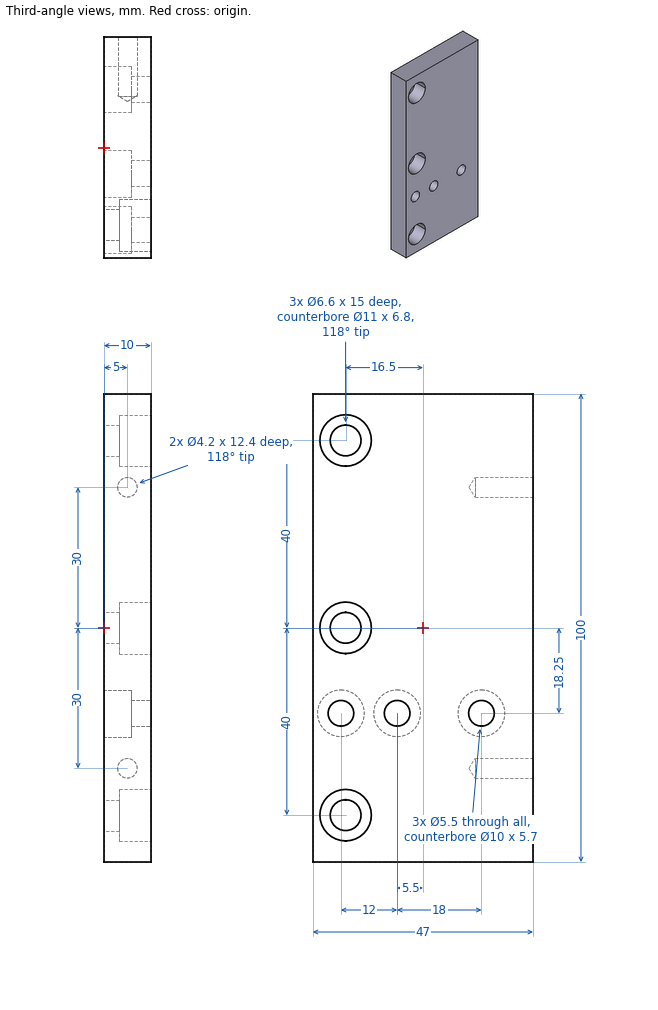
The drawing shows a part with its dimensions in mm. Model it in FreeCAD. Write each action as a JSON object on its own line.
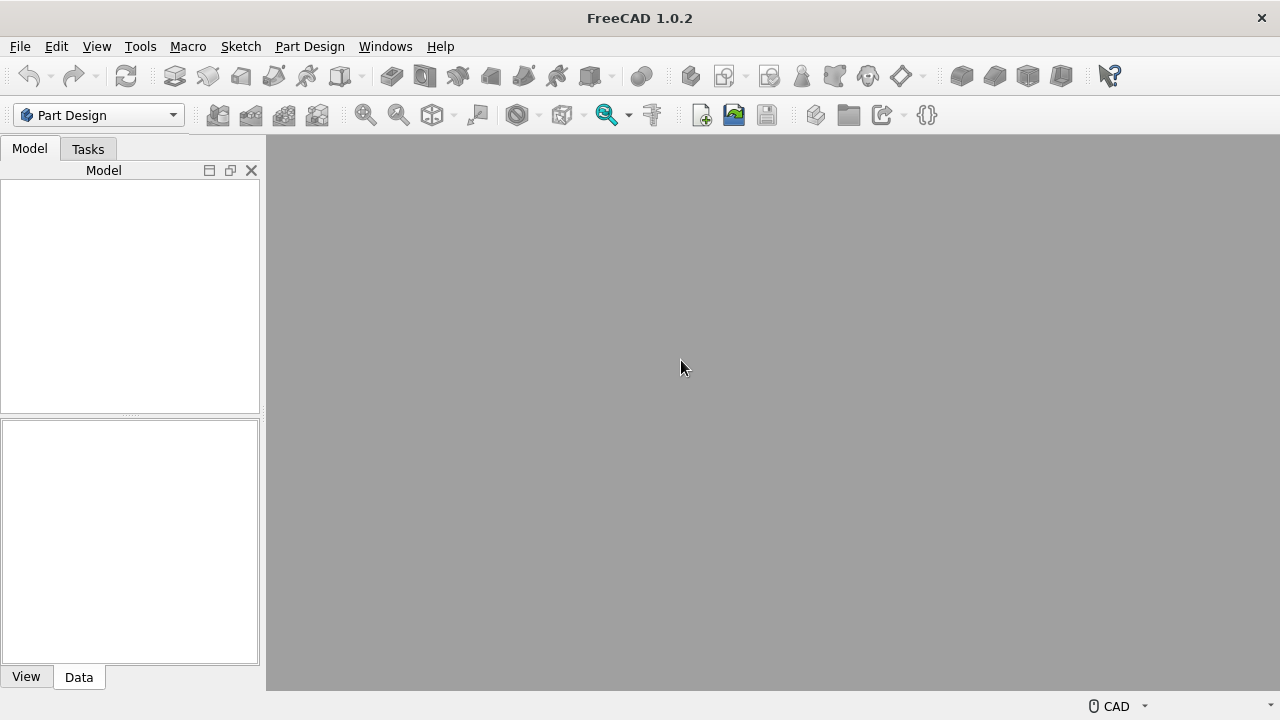
{"action": "left_click", "coordinate": [701, 116]}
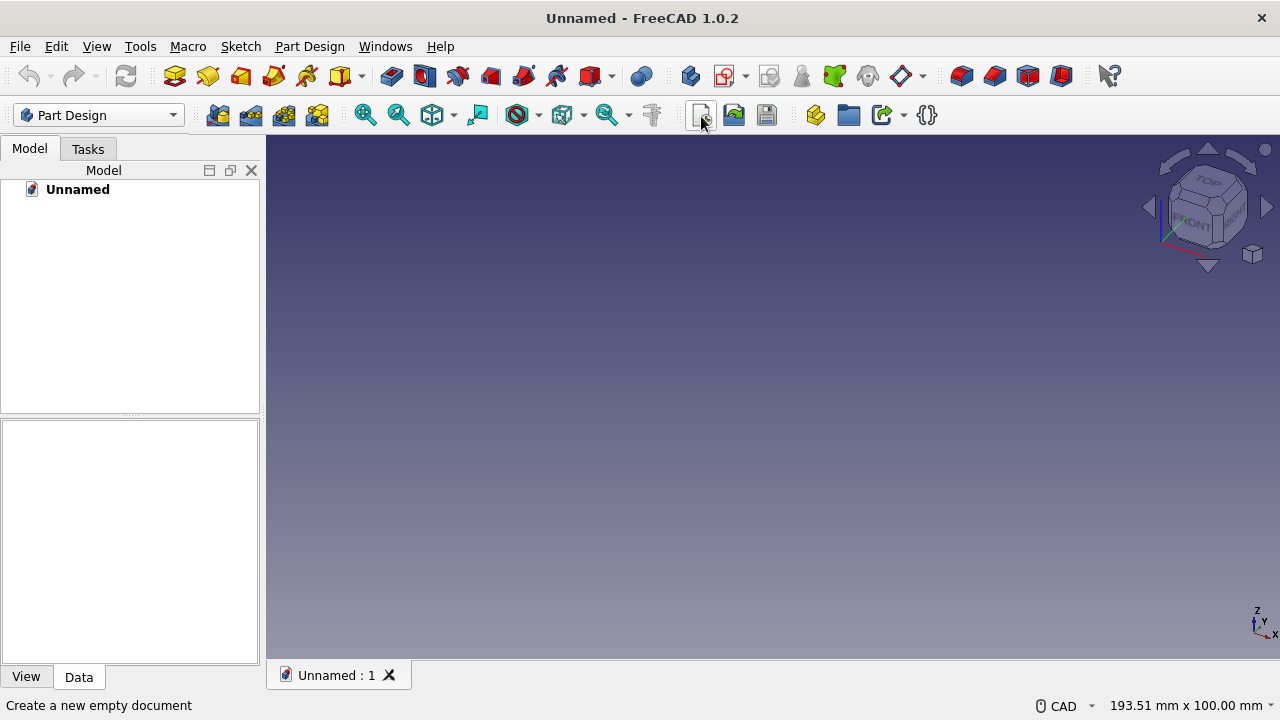
{"action": "left_click", "coordinate": [724, 76]}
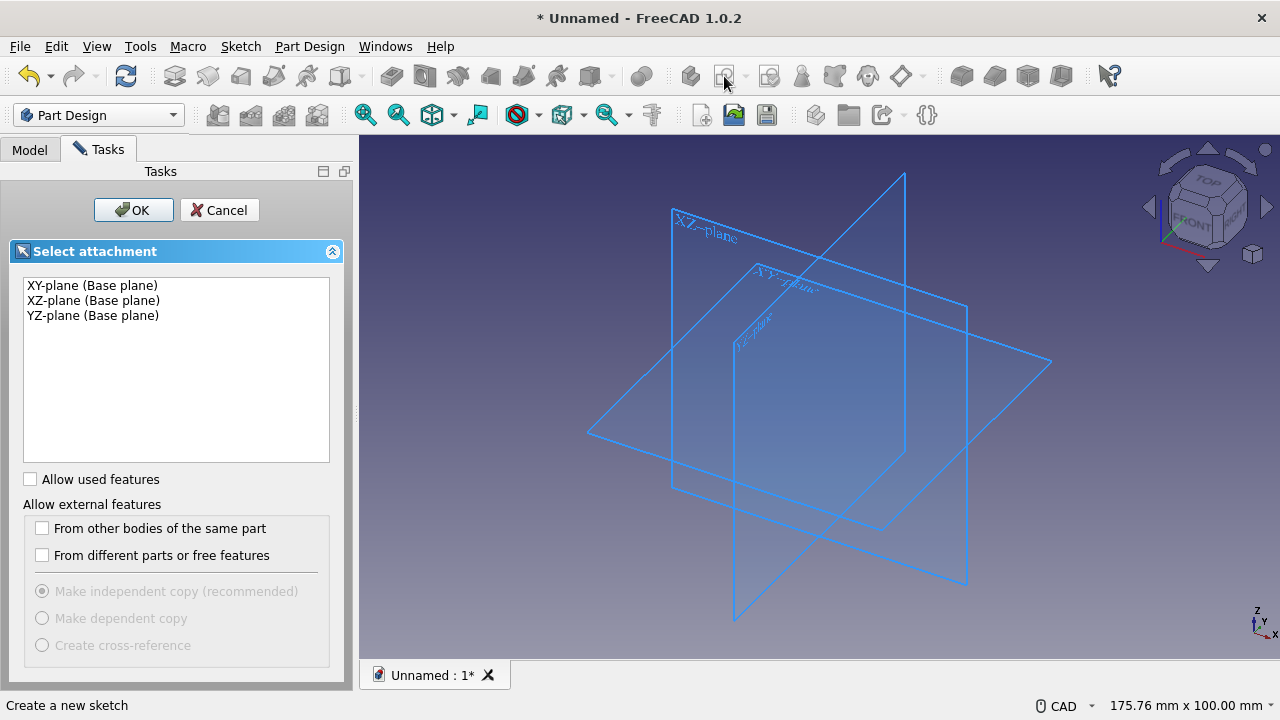
{"action": "left_click", "coordinate": [84, 316]}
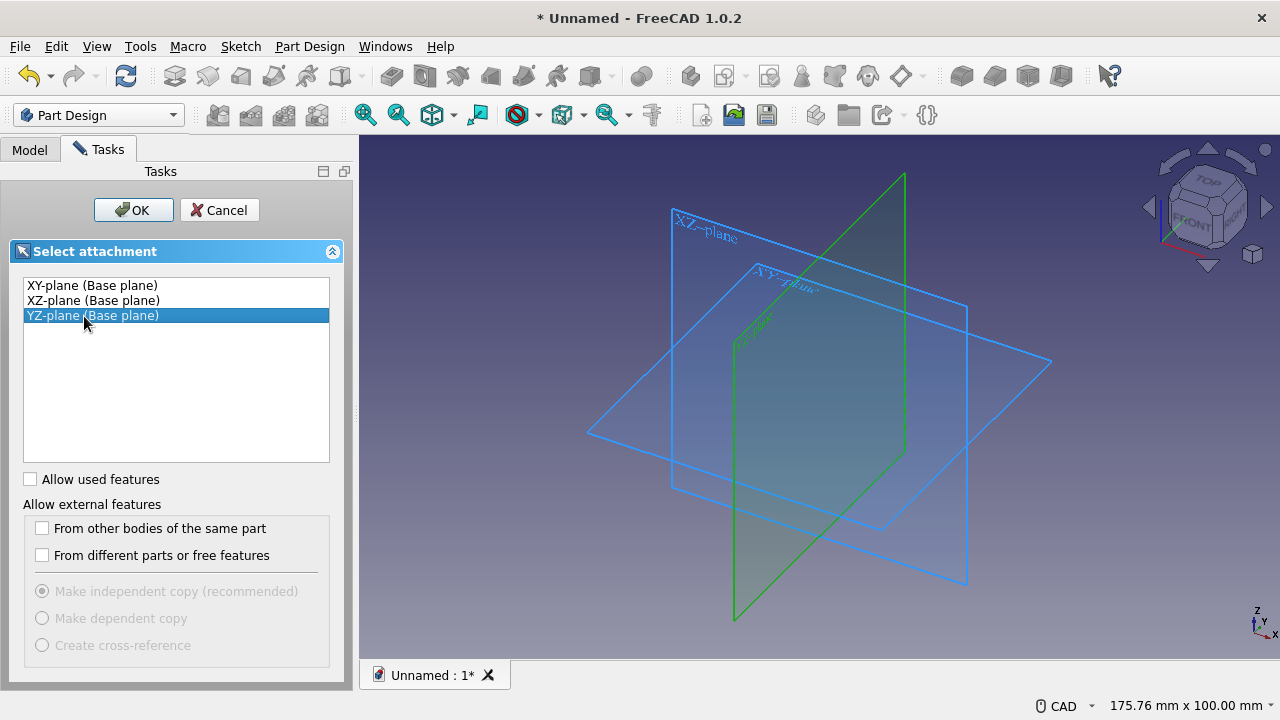
{"action": "left_click", "coordinate": [134, 210]}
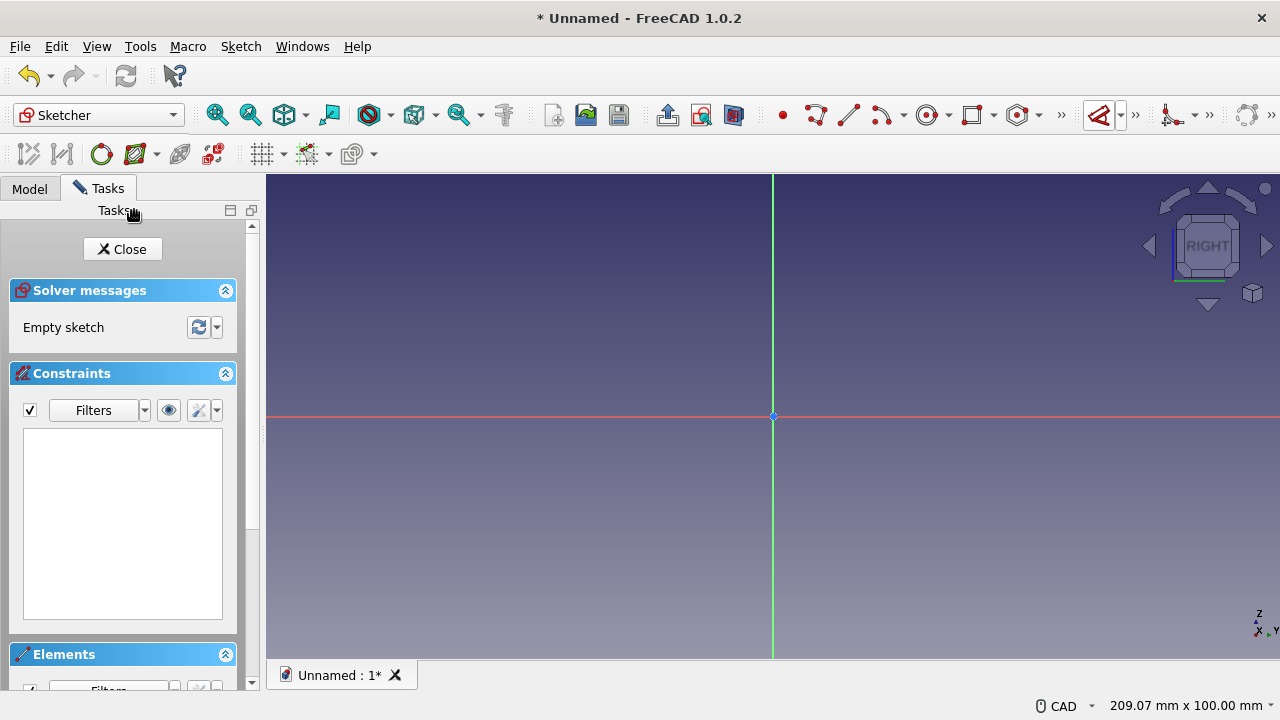
{"action": "scroll", "coordinate": [565, 416], "scroll_direction": "down", "scroll_amount": 2}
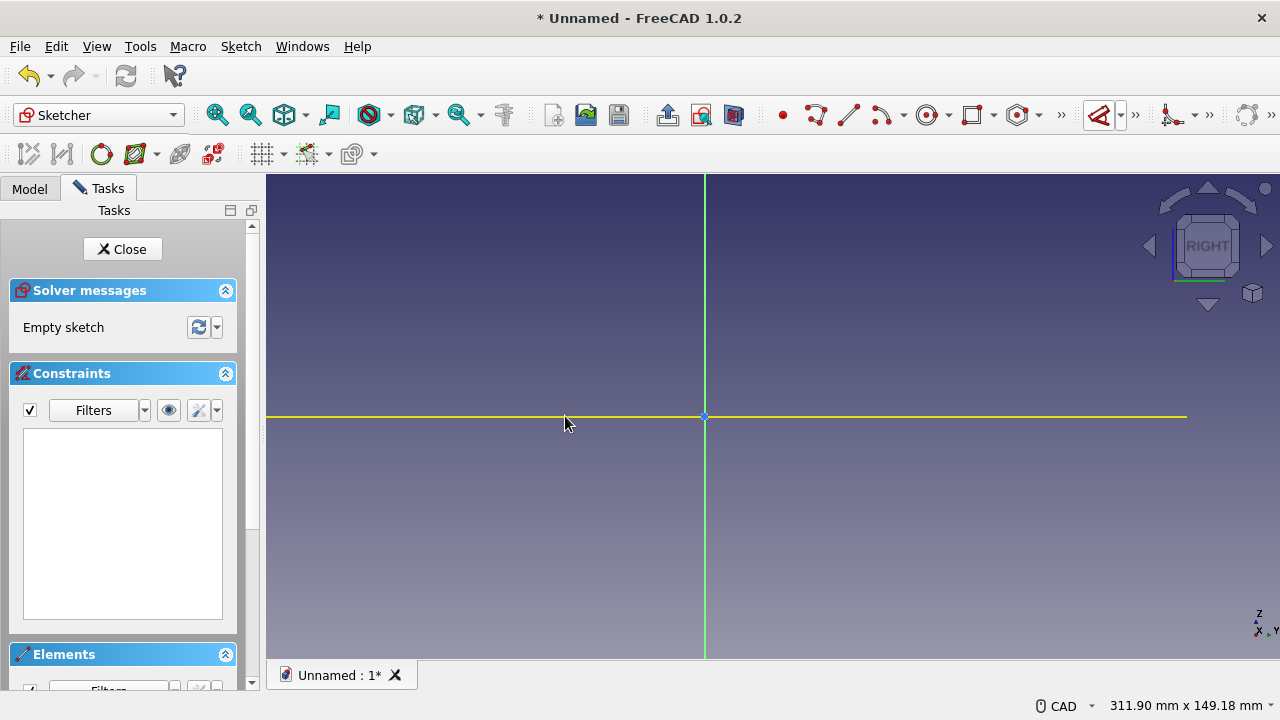
{"action": "key", "text": "g v"}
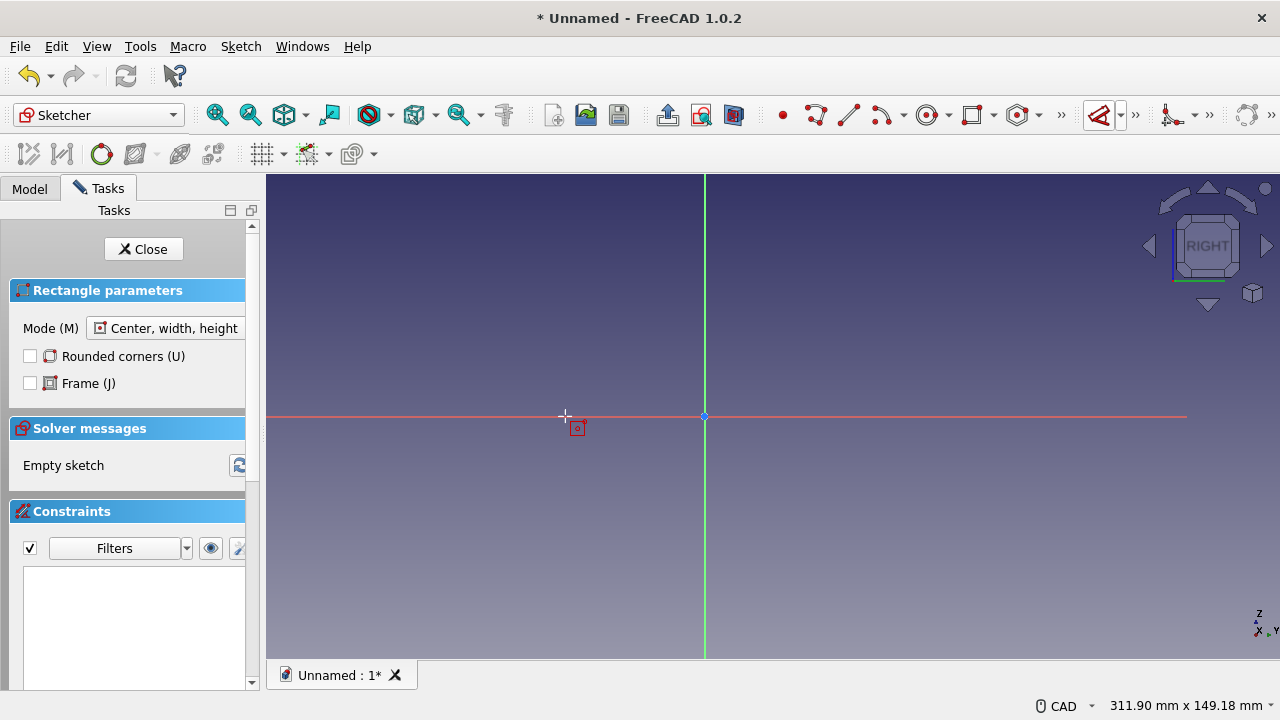
{"action": "left_click", "coordinate": [705, 416]}
{"action": "mouse_move", "coordinate": [781, 254]}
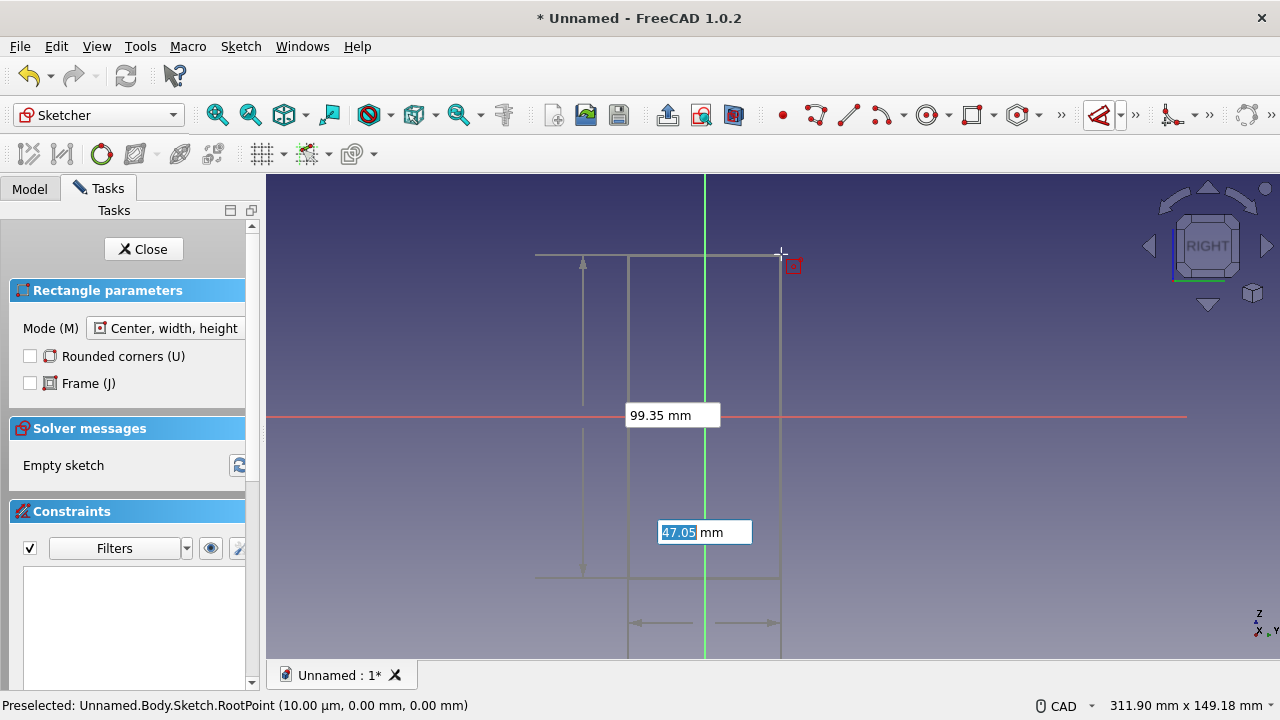
{"action": "type", "text": "47"}
{"action": "key", "text": "Tab"}
{"action": "type", "text": "100"}
{"action": "key", "text": "Return"}
{"action": "key", "text": "Escape"}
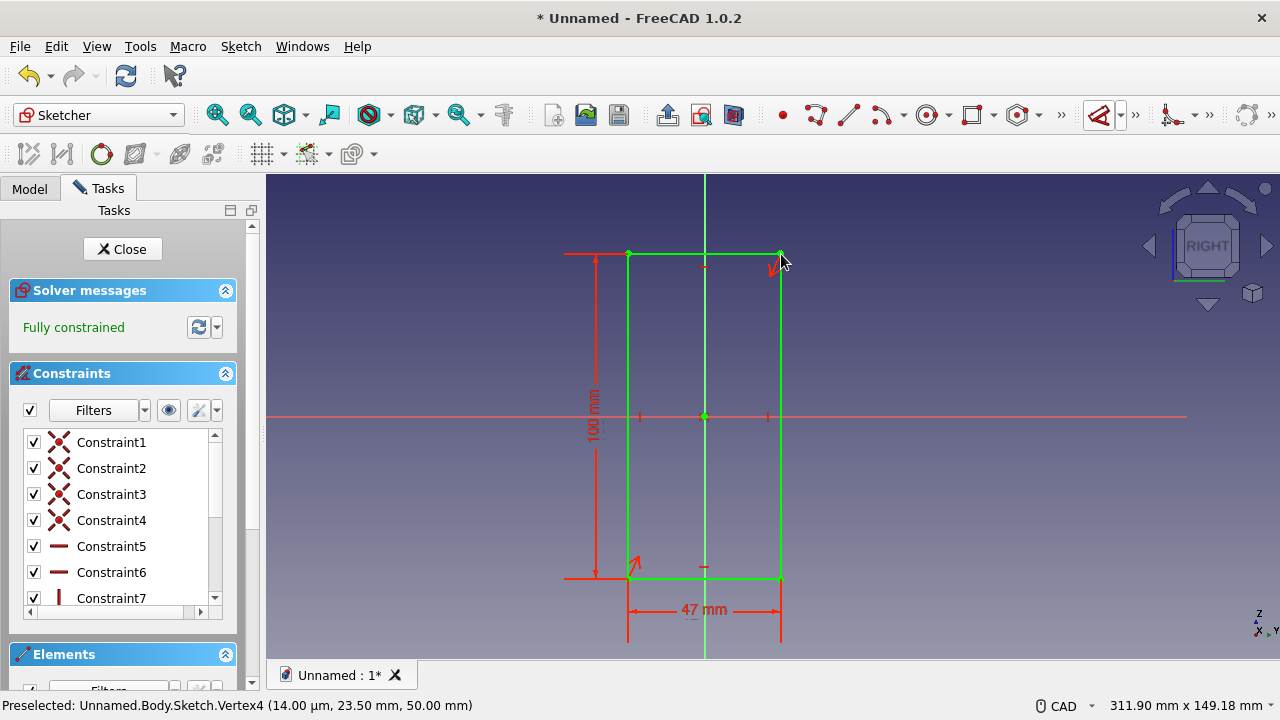
{"action": "left_click", "coordinate": [123, 249]}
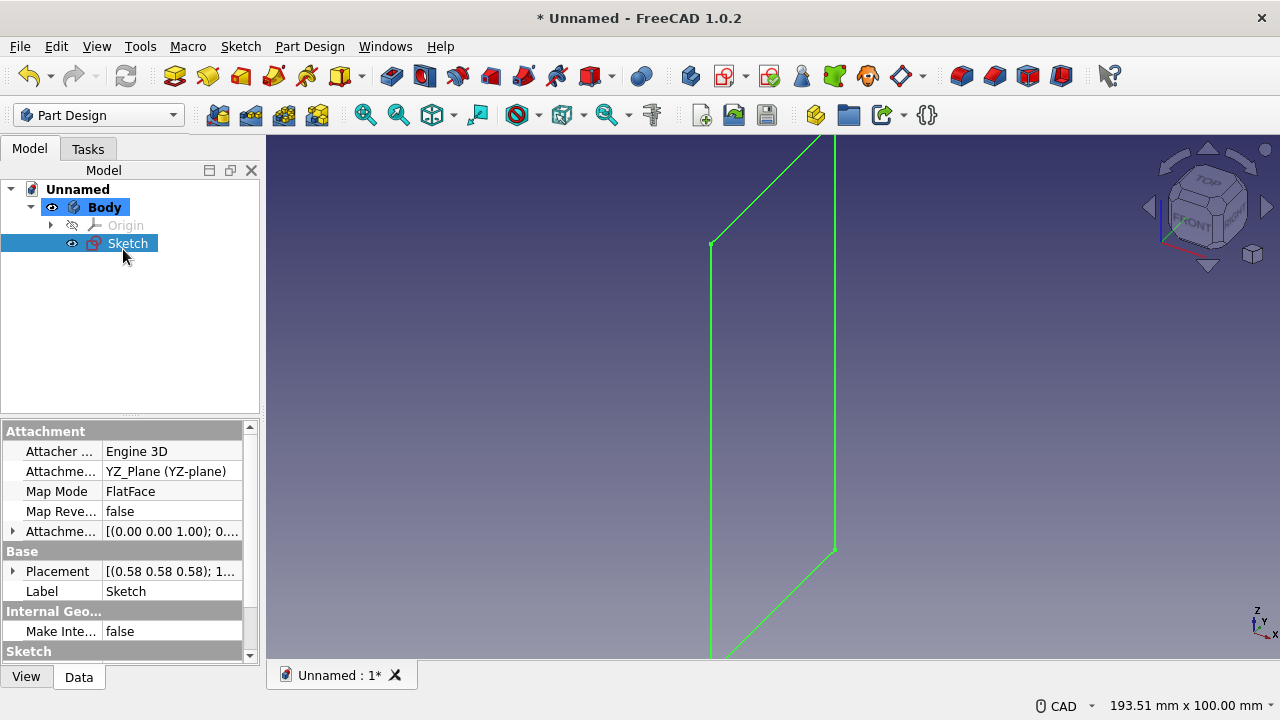
{"action": "left_click", "coordinate": [175, 76]}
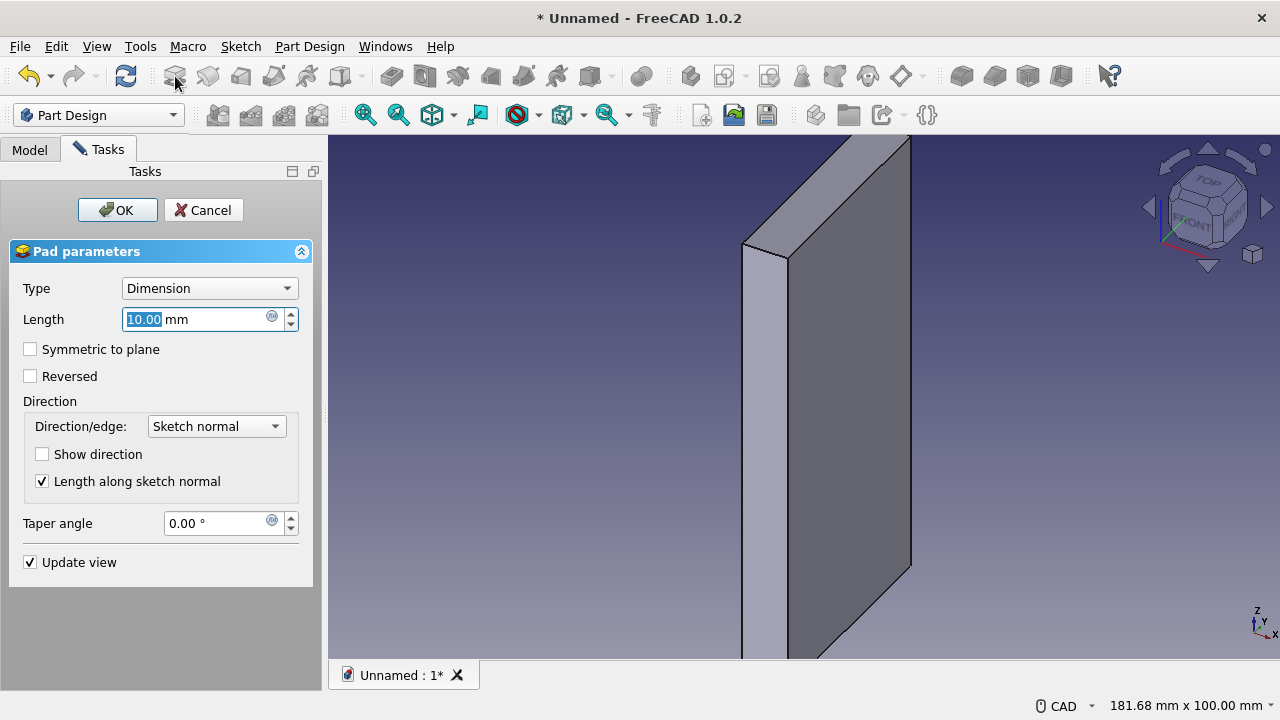
{"action": "type", "text": "10"}
{"action": "key", "text": "Tab"}